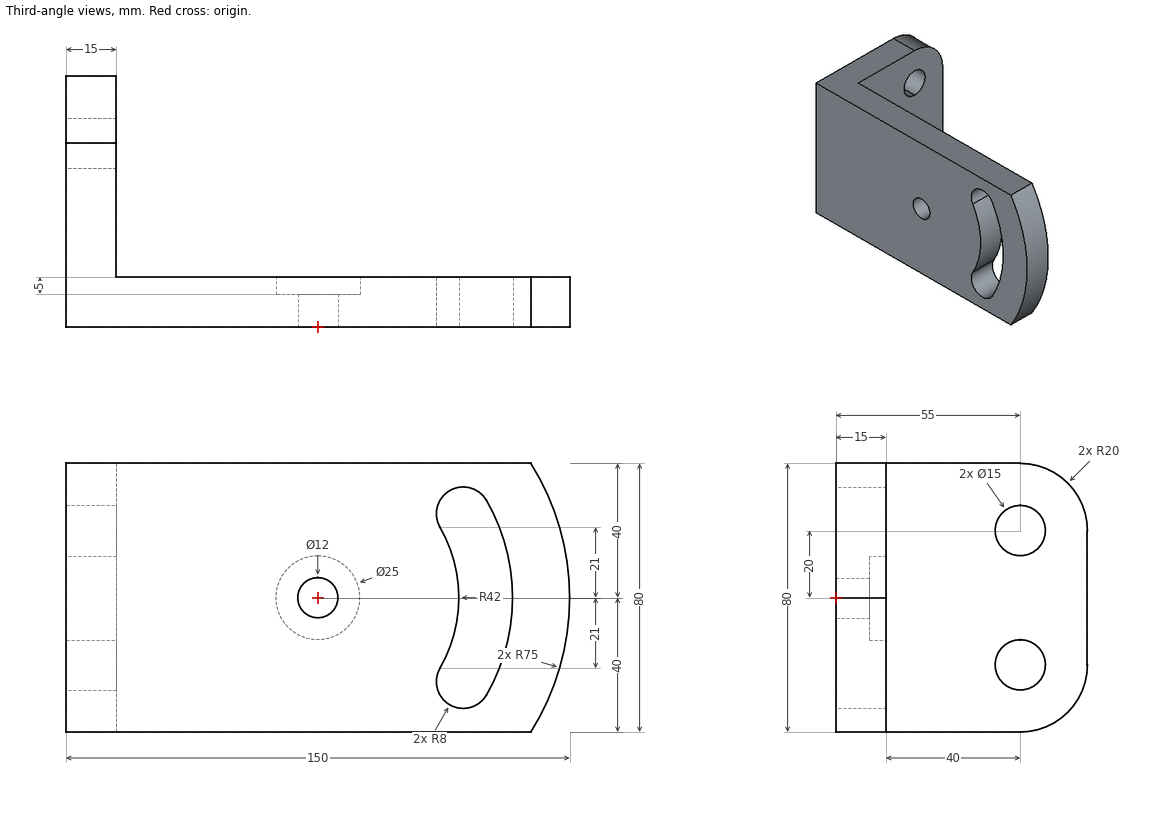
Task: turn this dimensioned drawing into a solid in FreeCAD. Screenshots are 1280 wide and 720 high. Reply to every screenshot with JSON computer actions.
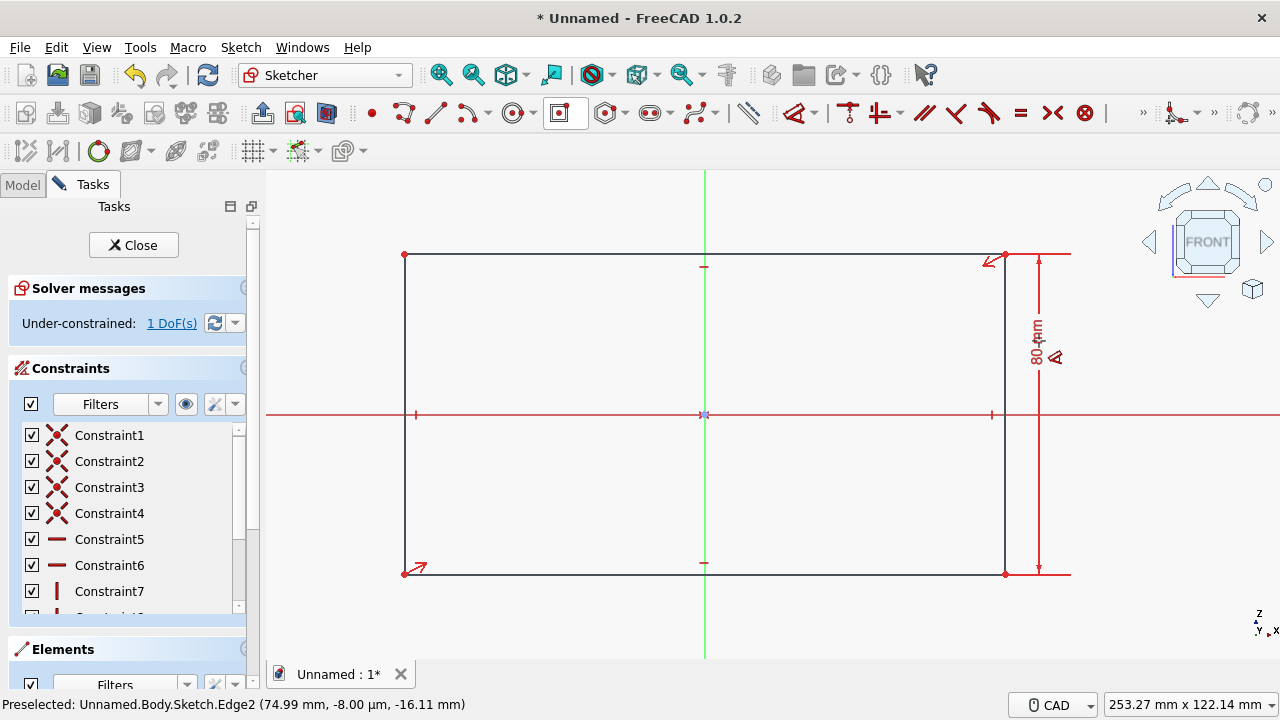
{"action": "left_click", "coordinate": [585, 575]}
{"action": "left_click", "coordinate": [567, 609]}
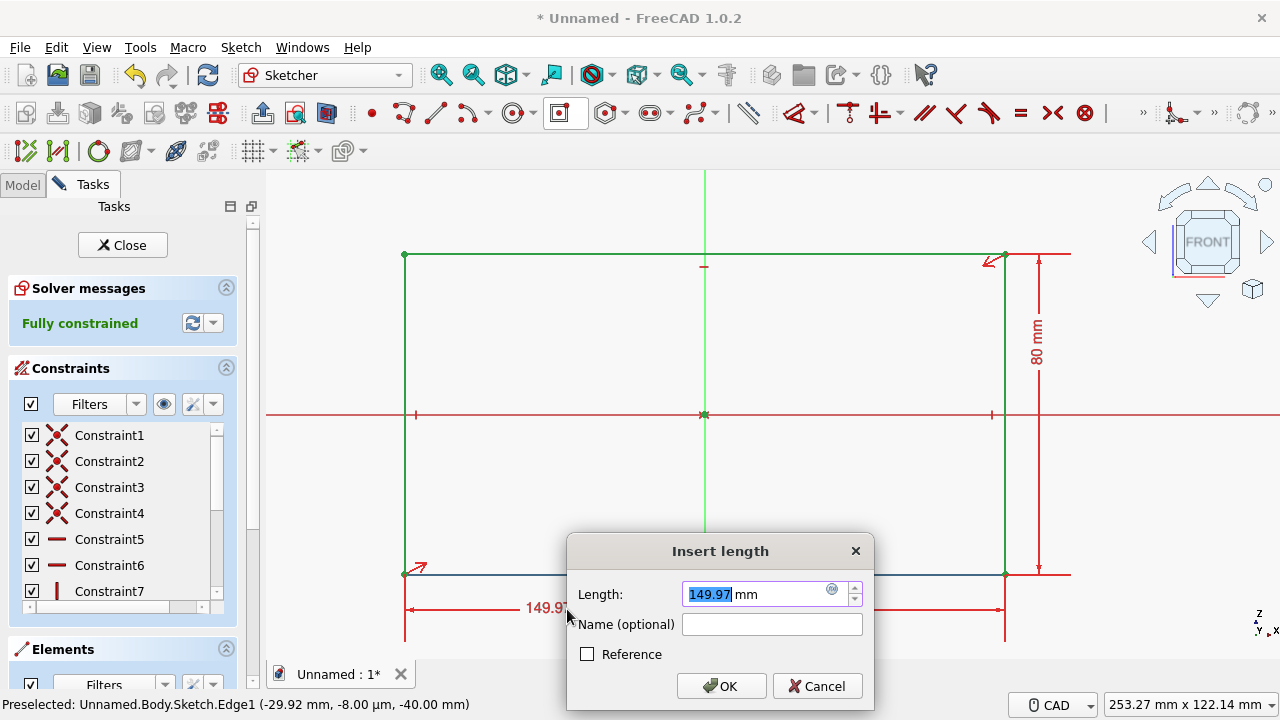
{"action": "type", "text": "150"}
{"action": "key", "text": "Return"}
{"action": "key", "text": "Escape"}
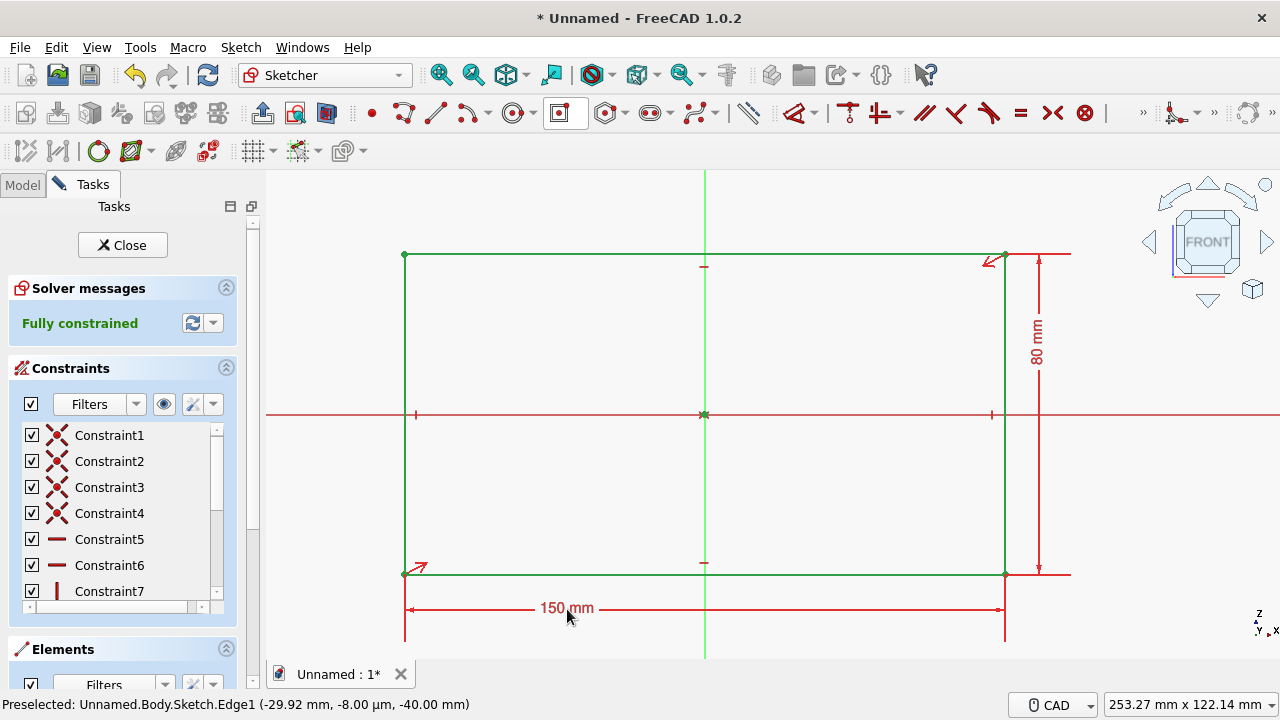
{"action": "left_click", "coordinate": [123, 245]}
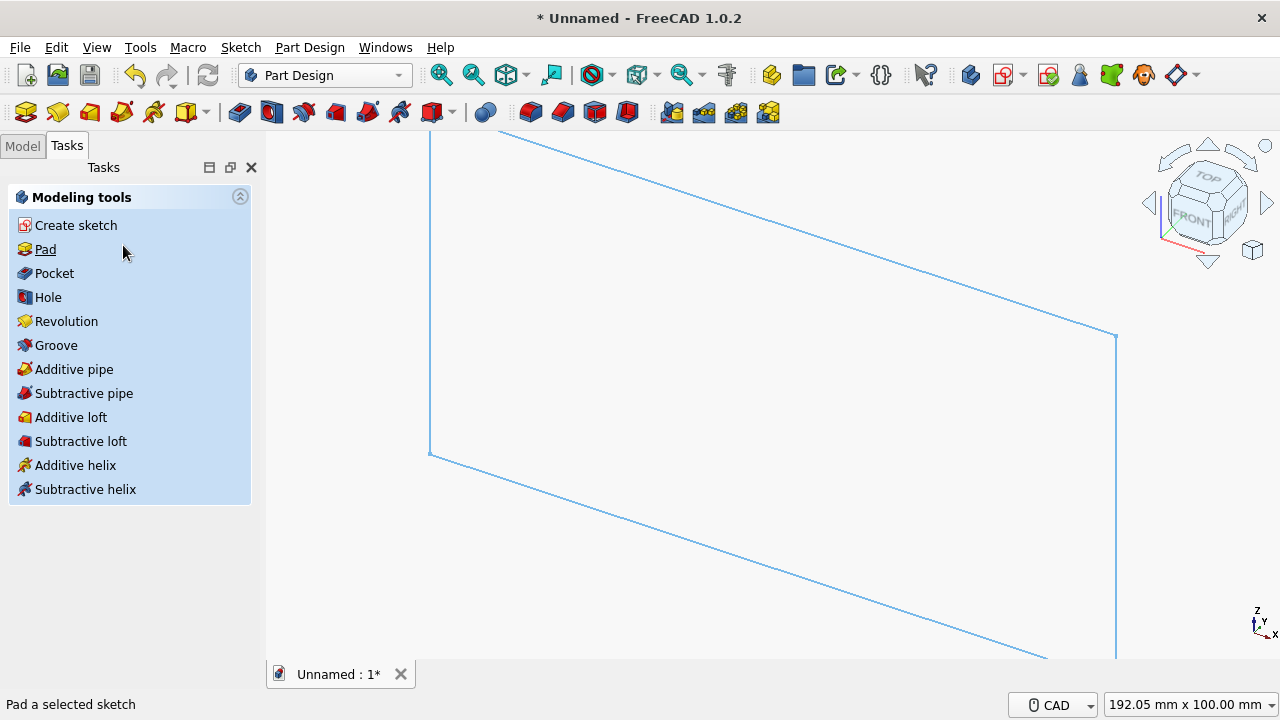
{"action": "left_click", "coordinate": [26, 112]}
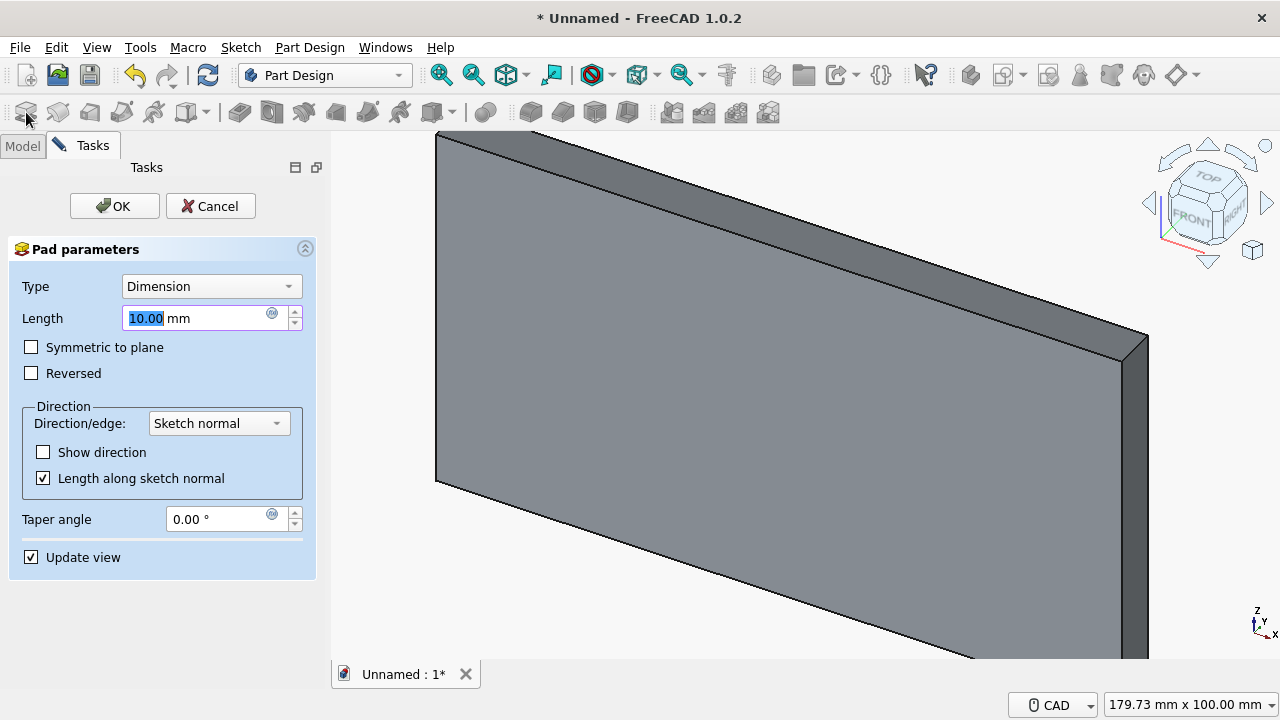
{"action": "type", "text": "15"}
{"action": "key", "text": "Tab"}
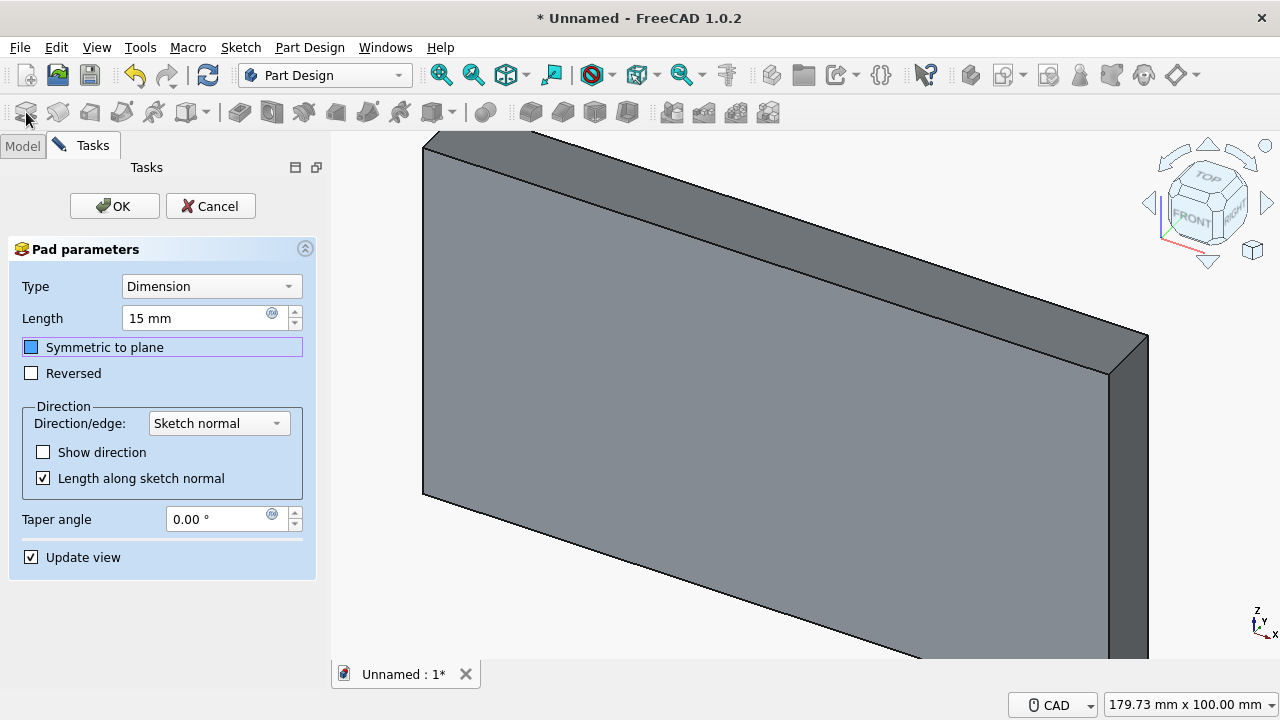
{"action": "left_click", "coordinate": [30, 373]}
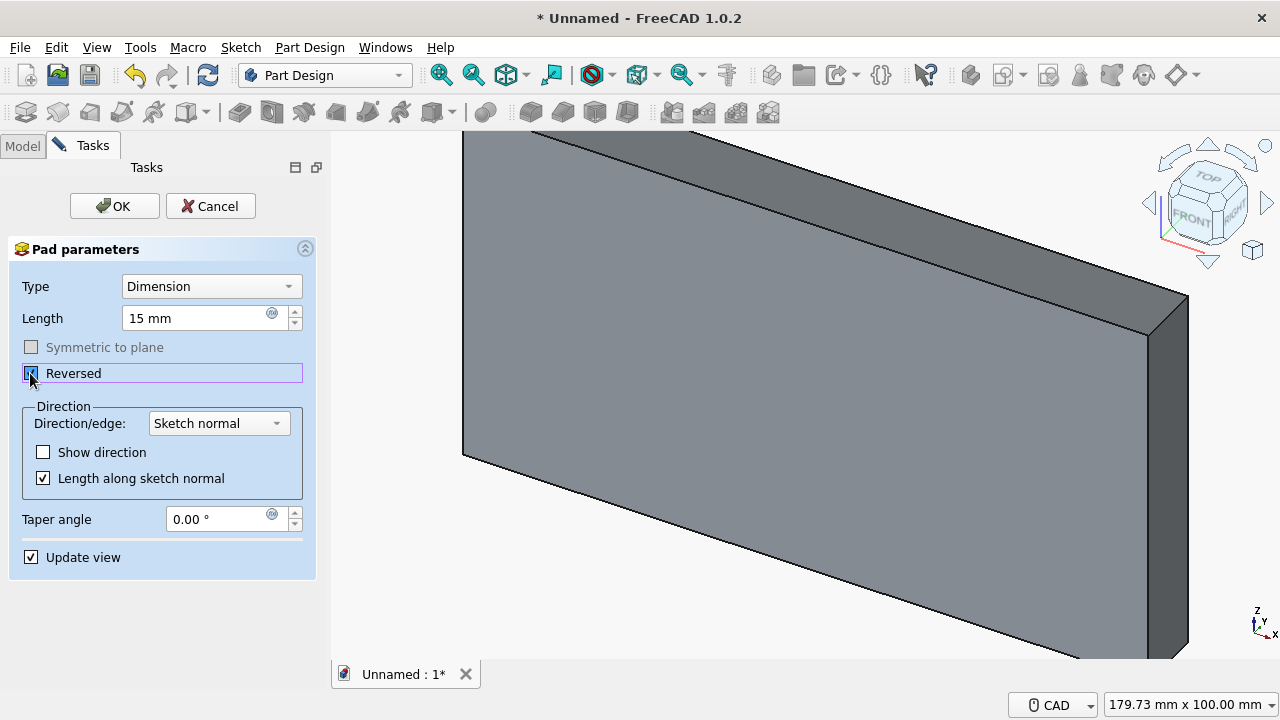
{"action": "left_click", "coordinate": [115, 206]}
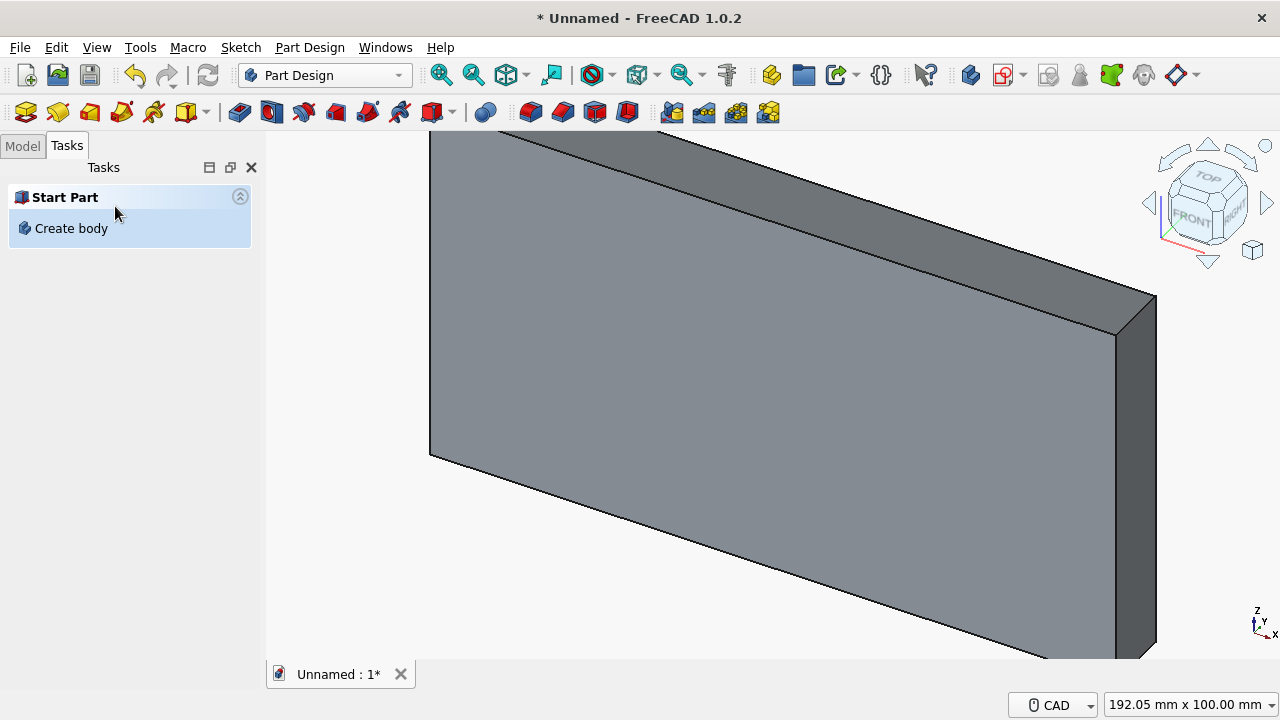
{"action": "left_click", "coordinate": [442, 76]}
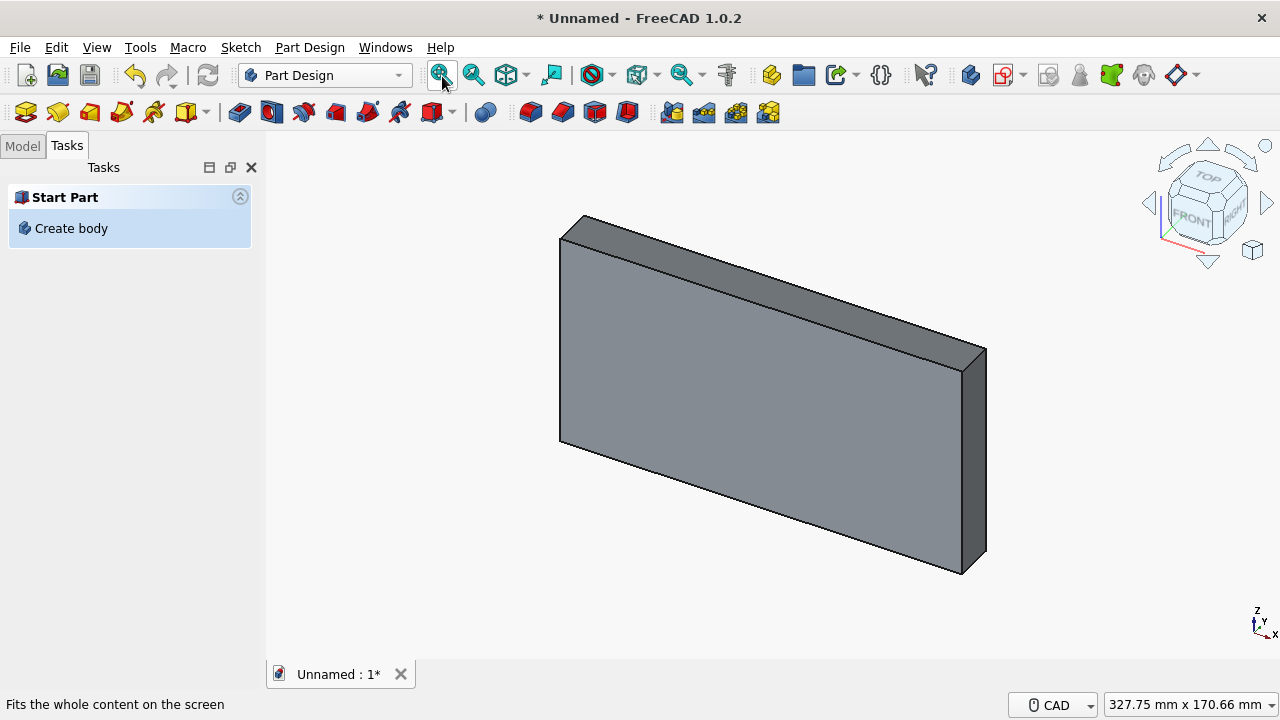
{"action": "key", "text": "4"}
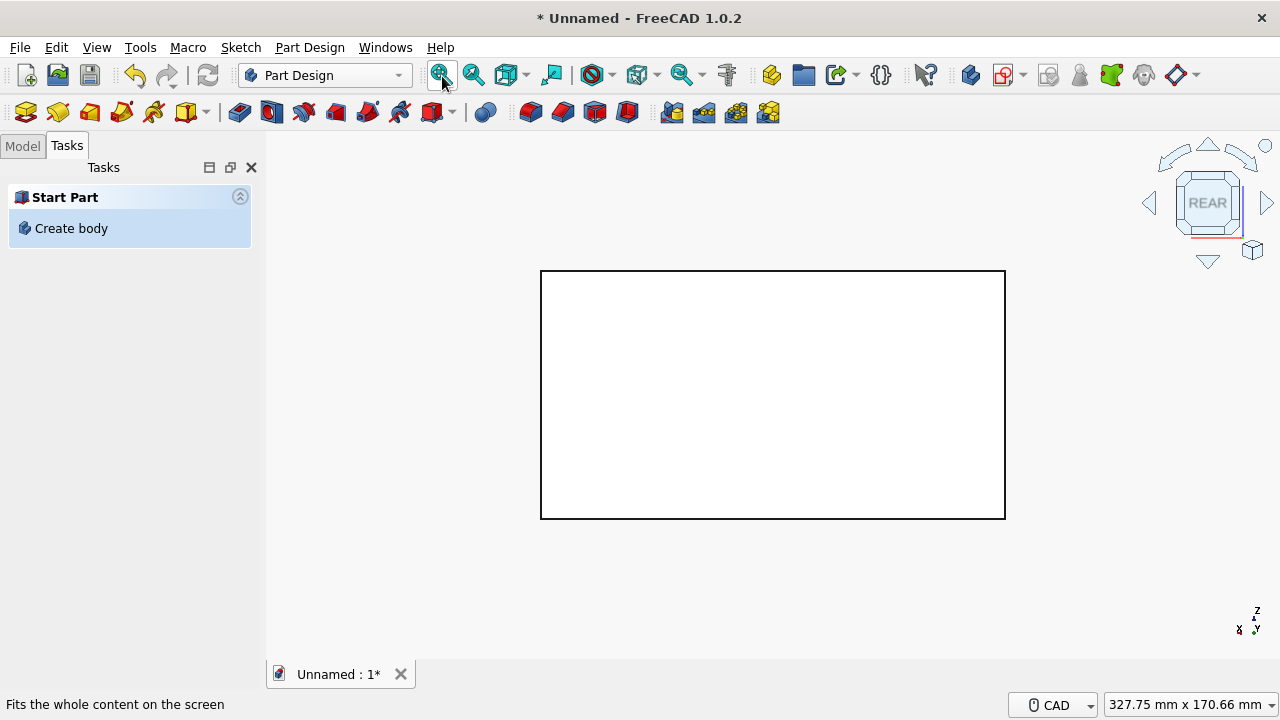
{"action": "left_click", "coordinate": [707, 394]}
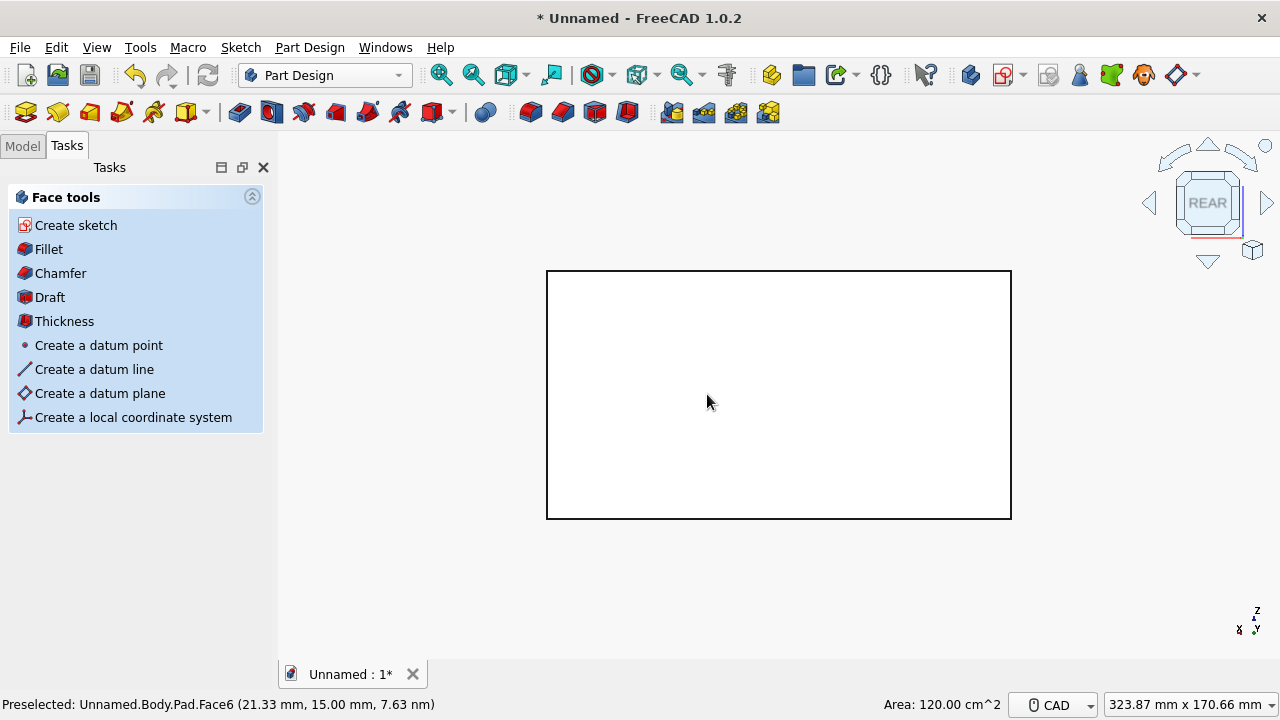
{"action": "left_click", "coordinate": [1004, 76]}